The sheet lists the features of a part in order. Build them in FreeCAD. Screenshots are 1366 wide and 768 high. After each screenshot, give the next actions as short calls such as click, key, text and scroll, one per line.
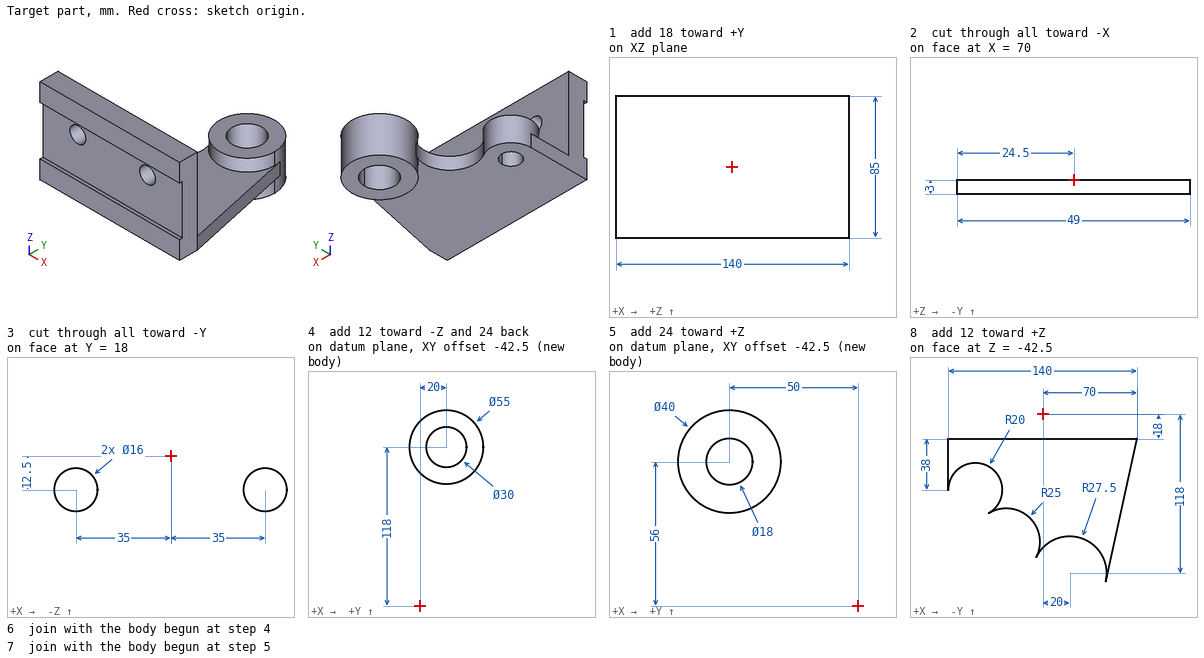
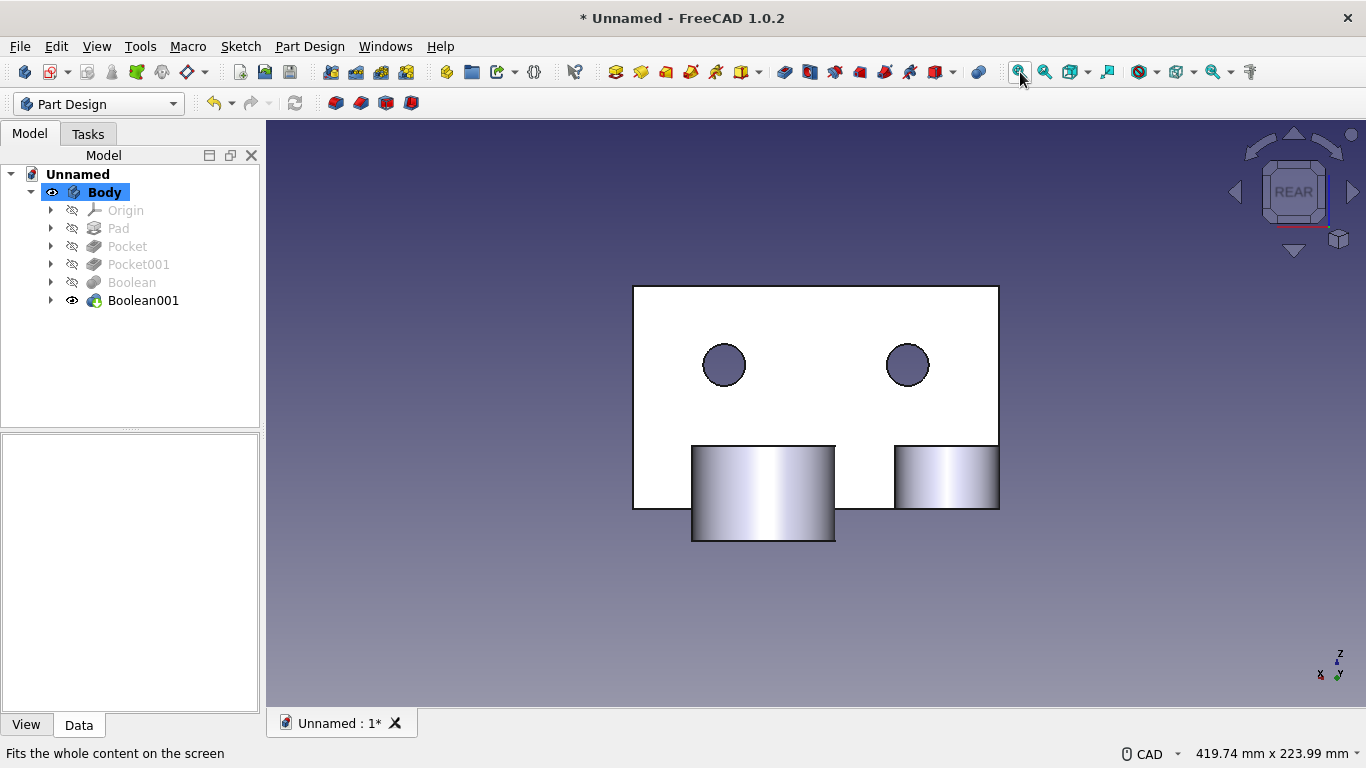
key(5)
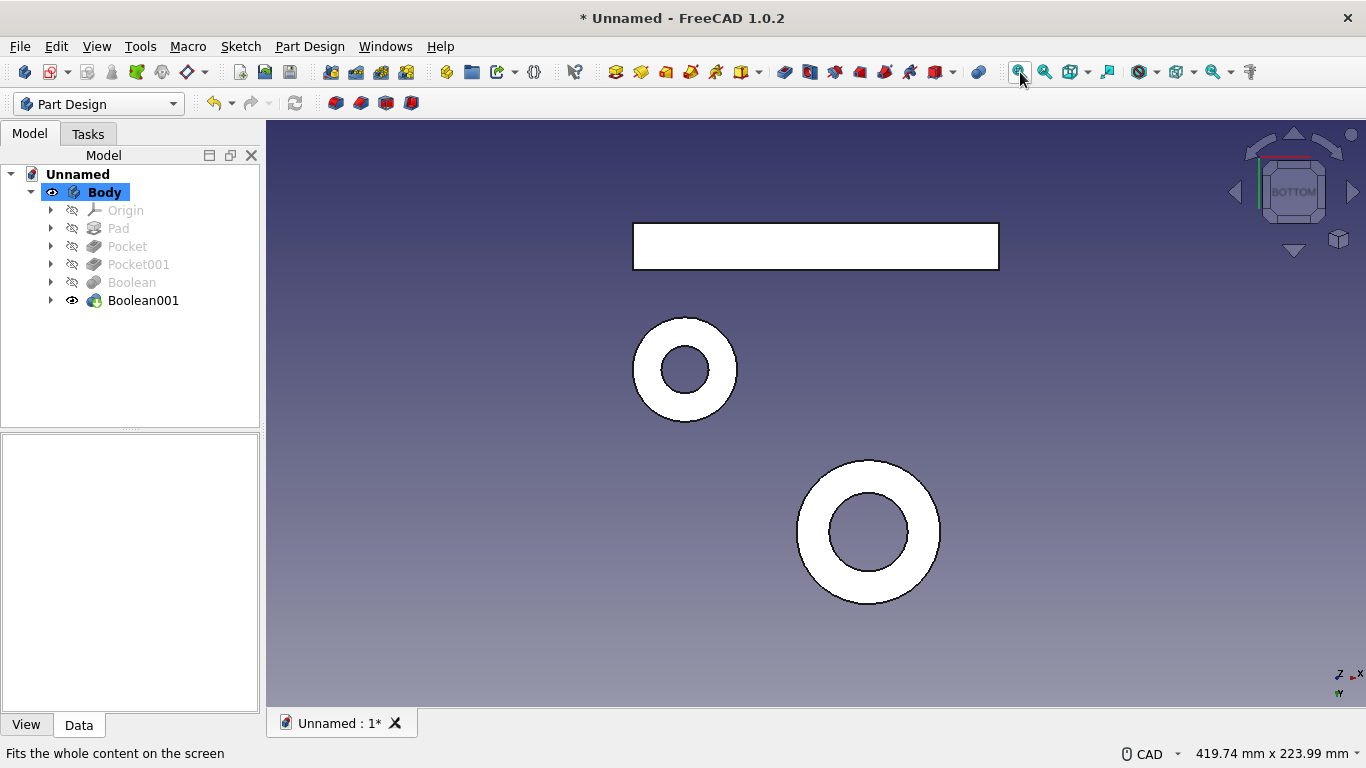
click(973, 245)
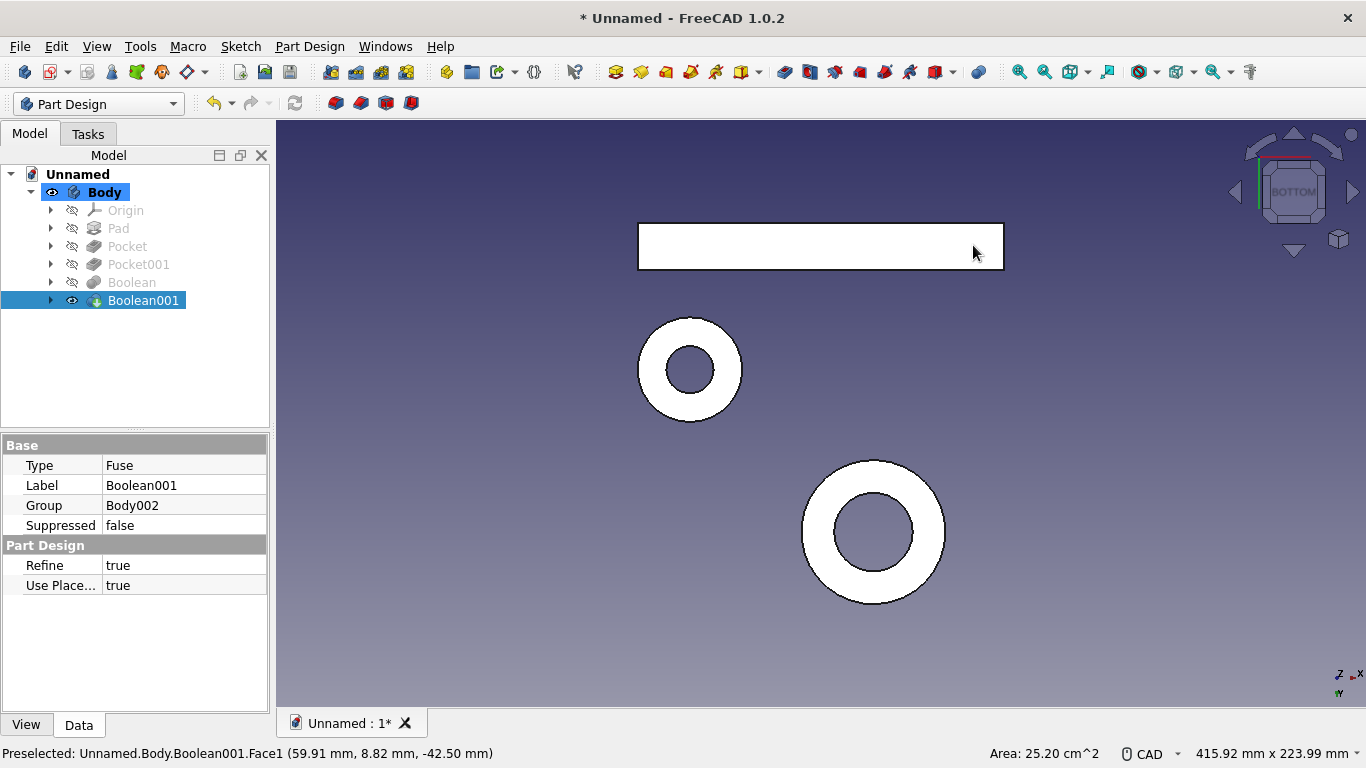
click(50, 72)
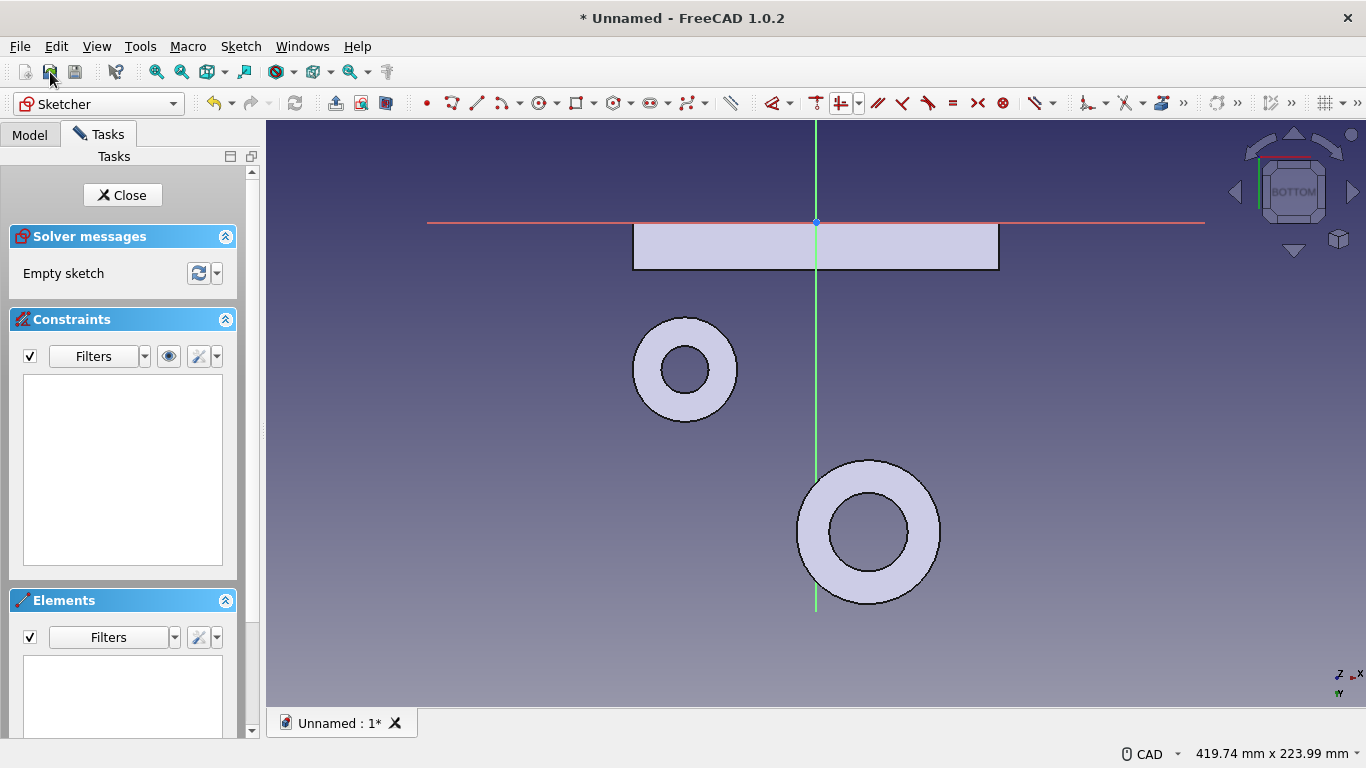
click(386, 104)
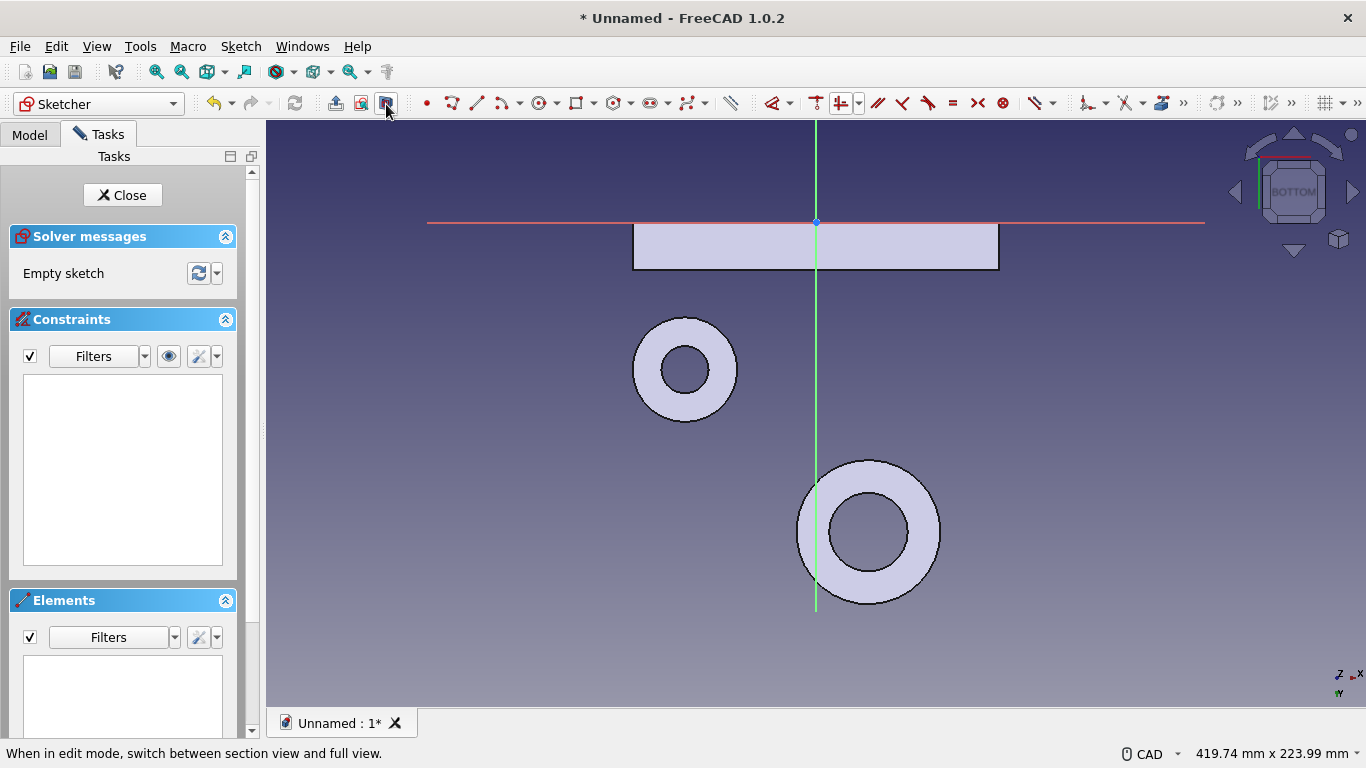
click(452, 104)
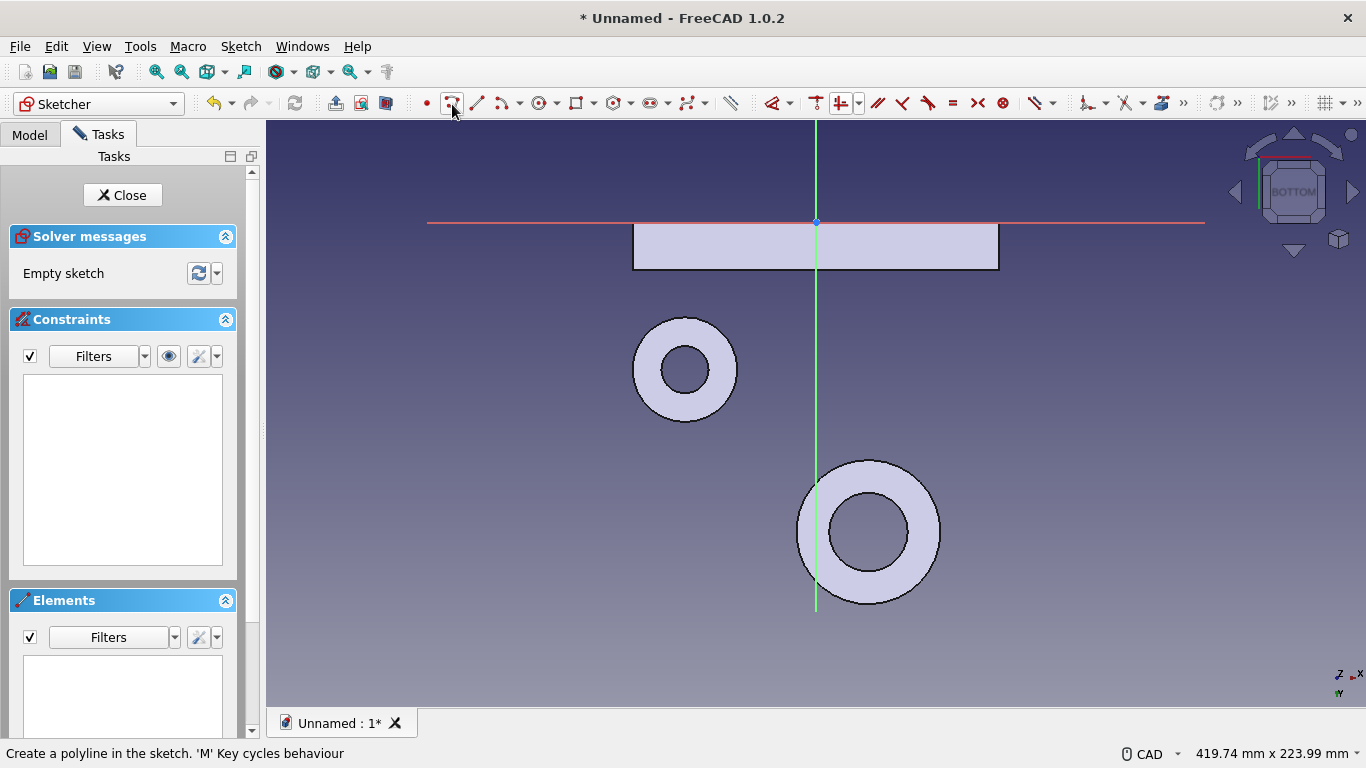
click(939, 548)
click(999, 270)
click(633, 270)
click(633, 370)
right_click(633, 370)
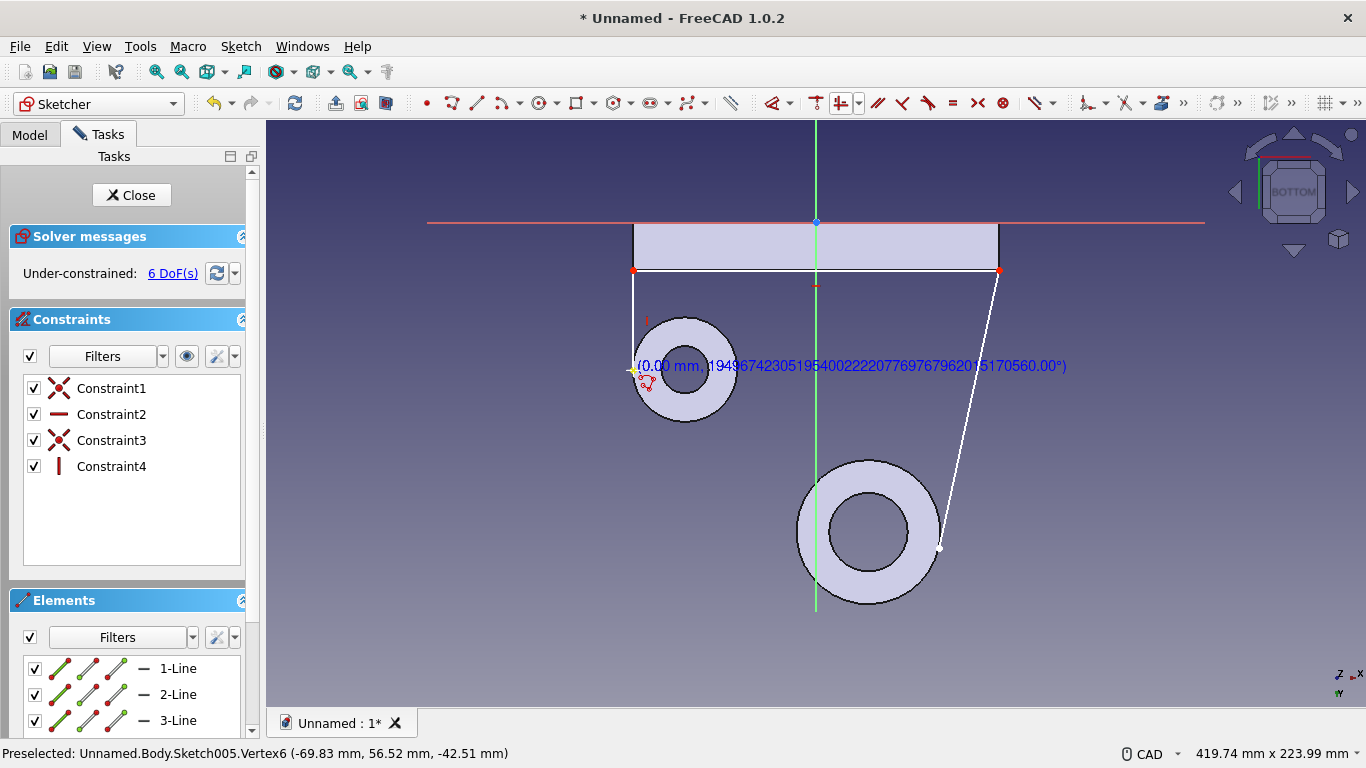
key(g)
key(3)
key(a)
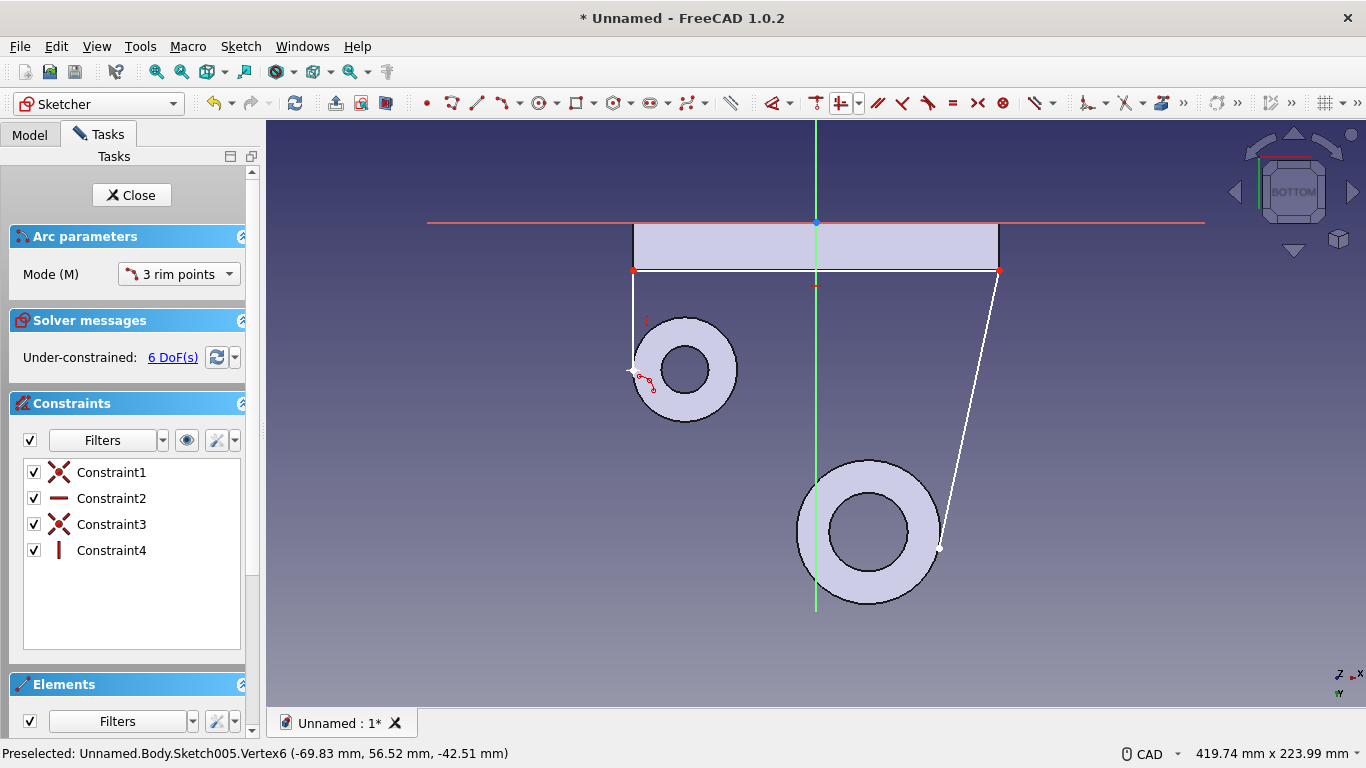
click(633, 371)
click(712, 415)
click(711, 324)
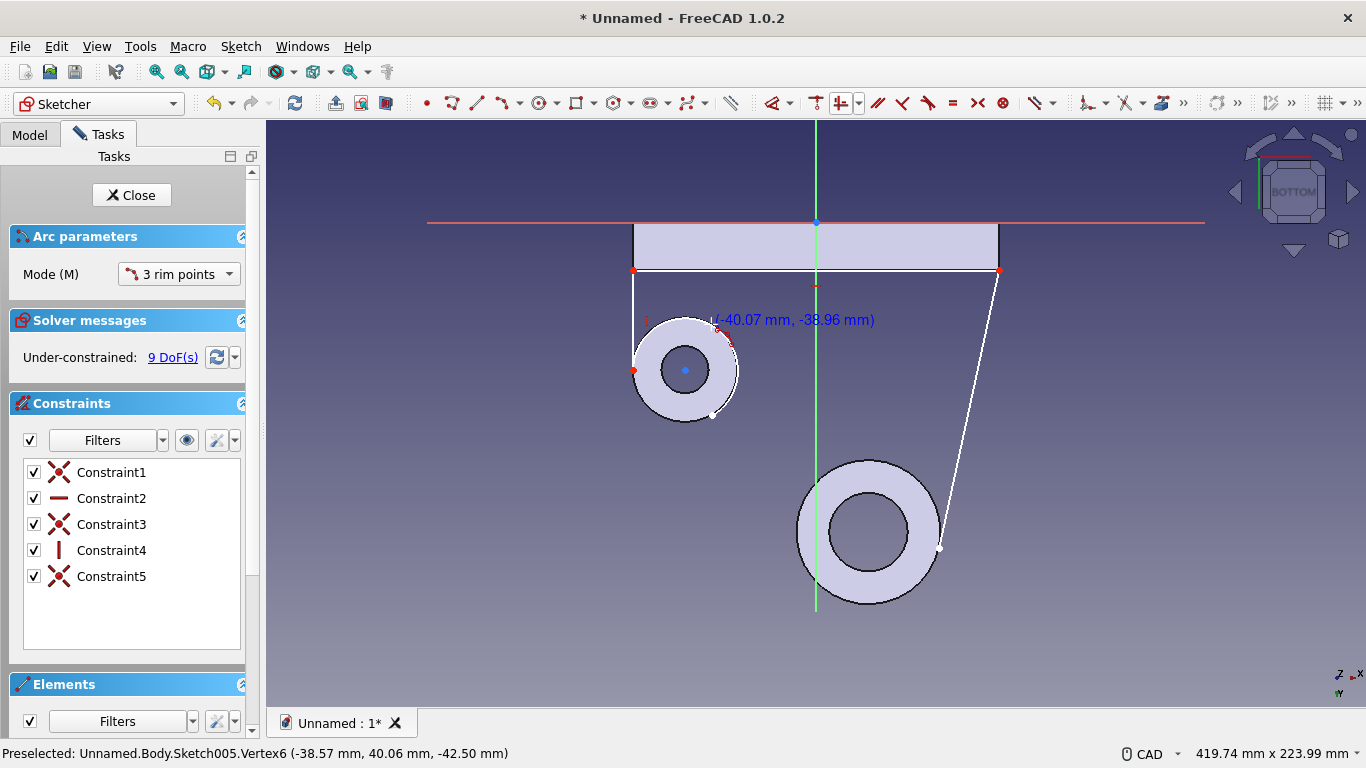
click(712, 416)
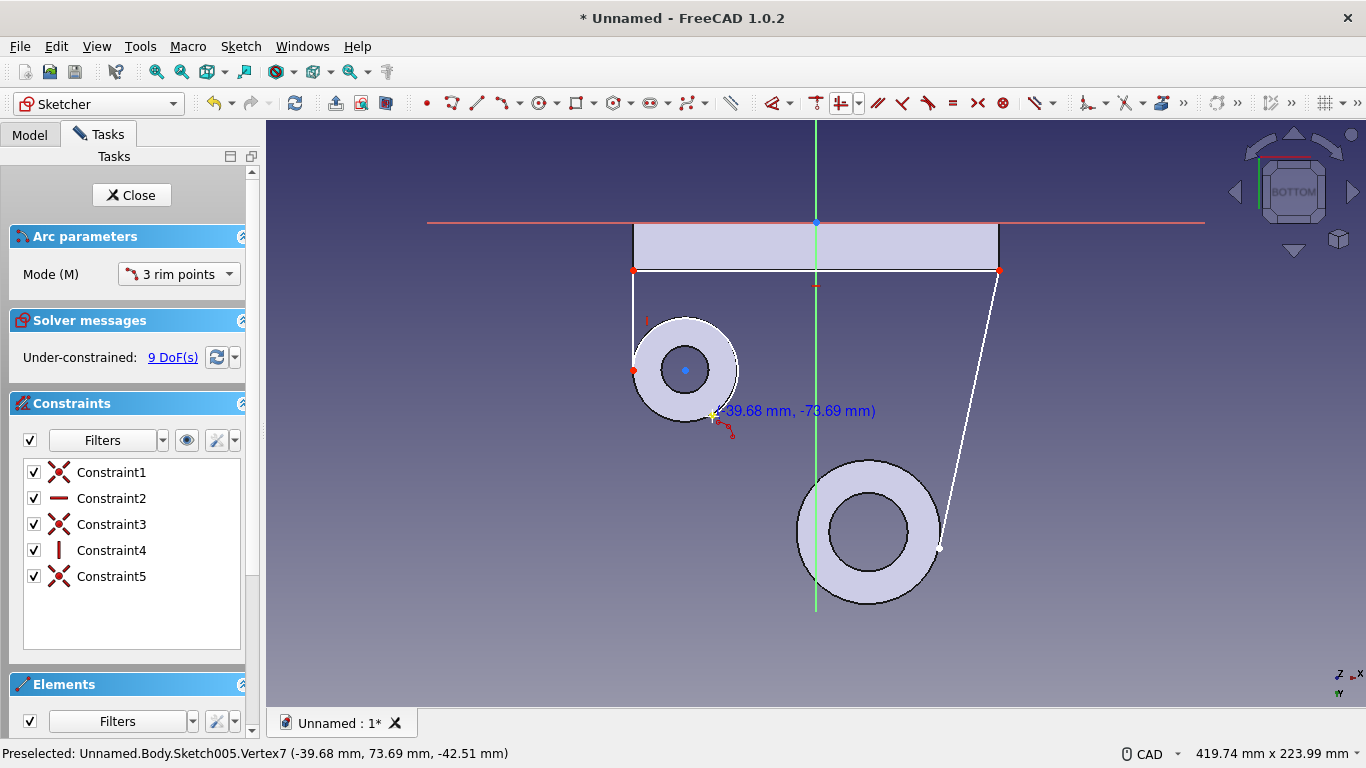
scroll(804, 500, up, 2)